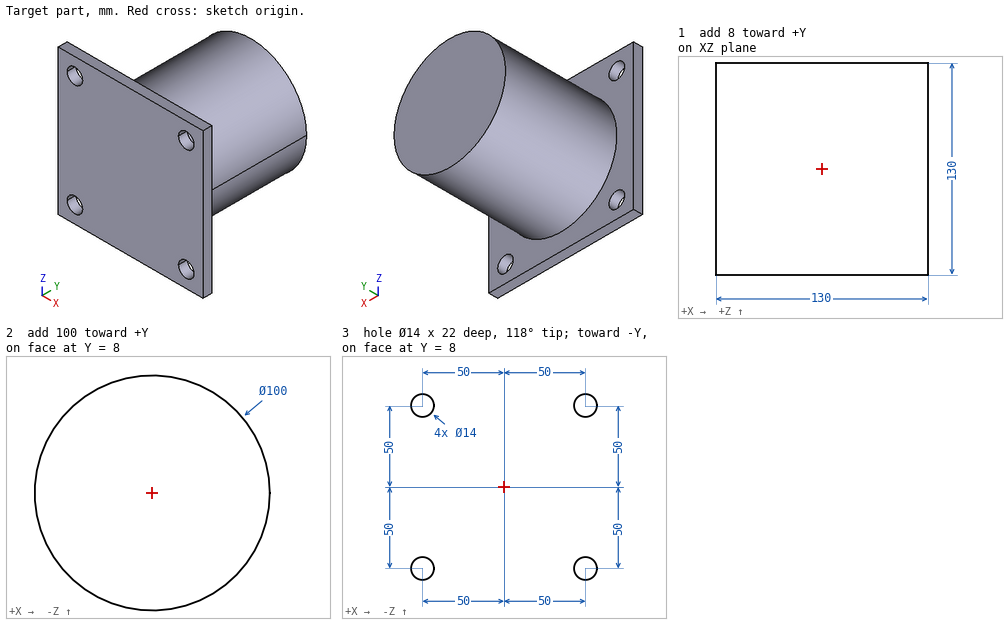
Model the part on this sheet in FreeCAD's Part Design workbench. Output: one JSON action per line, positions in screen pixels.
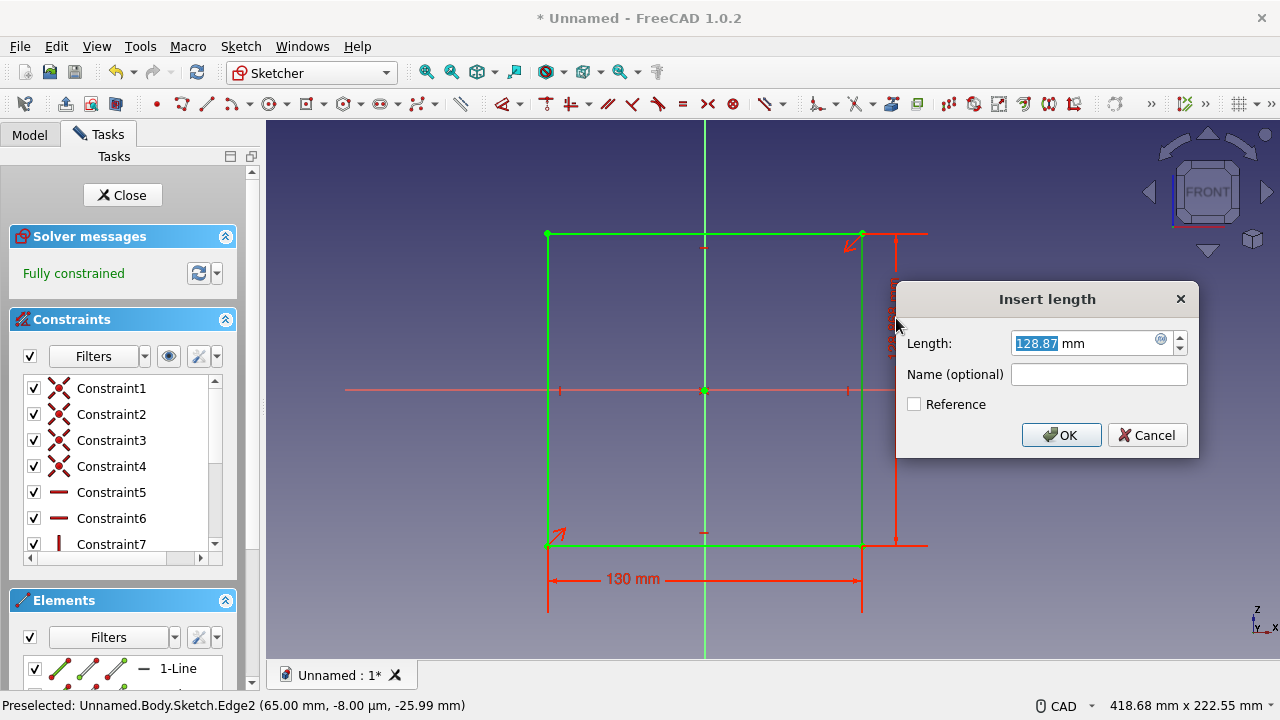
{"action": "type", "text": "130"}
{"action": "key", "text": "Return"}
{"action": "key", "text": "Escape"}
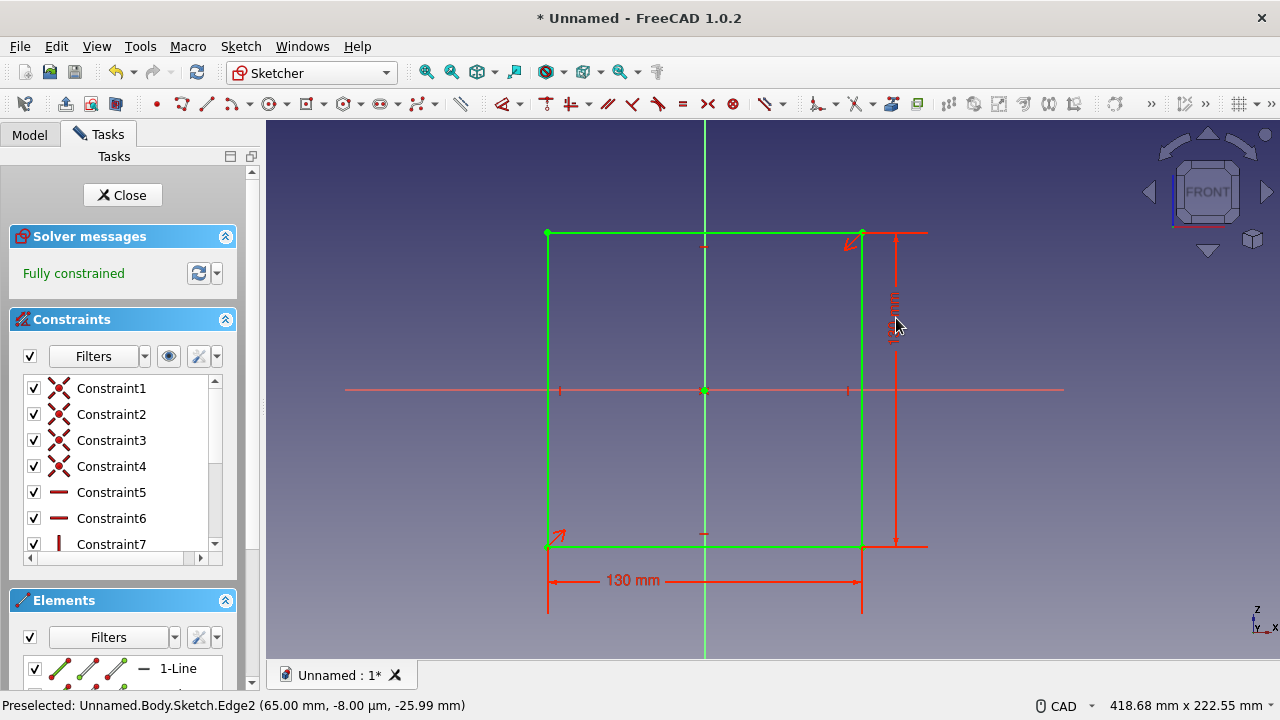
{"action": "left_click", "coordinate": [123, 195]}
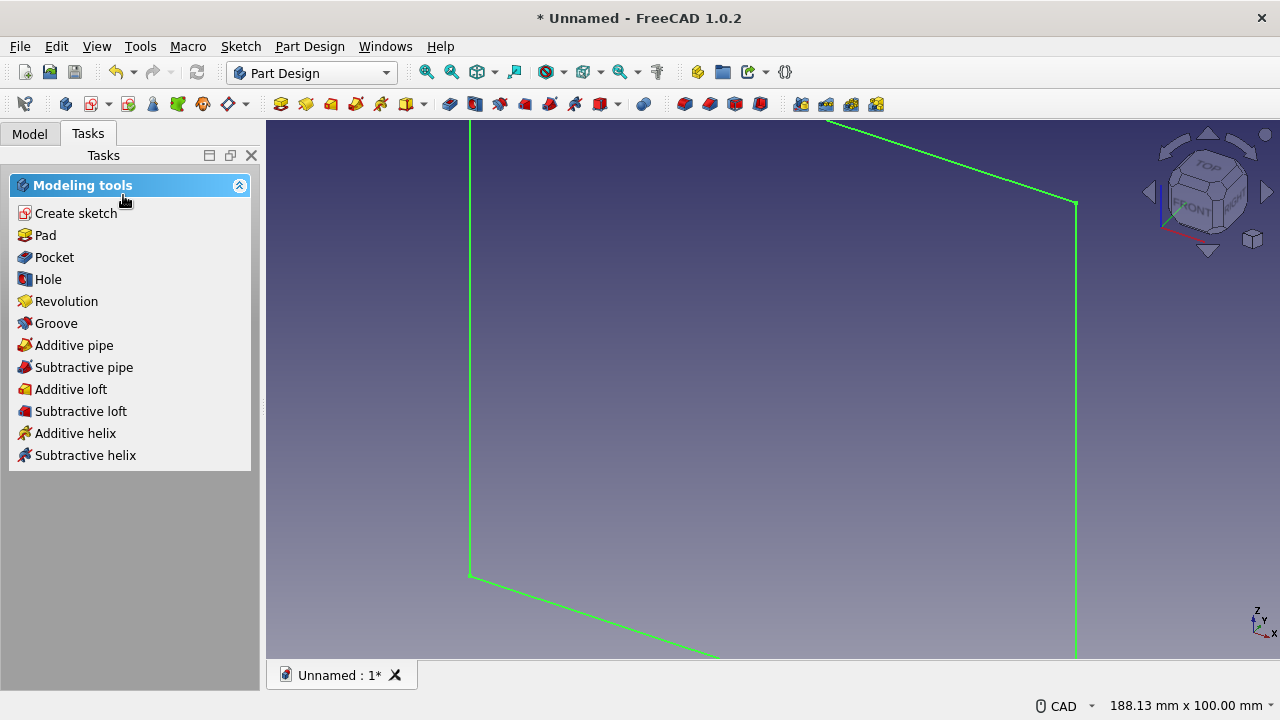
{"action": "left_click", "coordinate": [281, 104]}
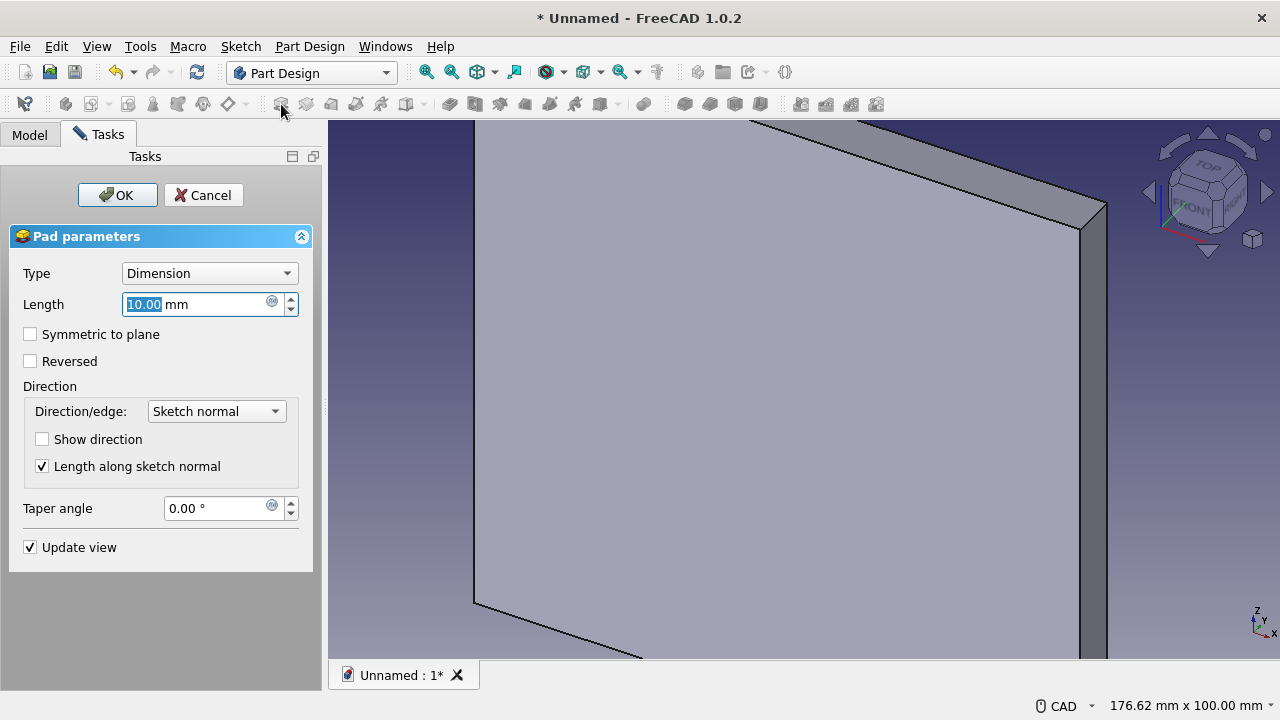
{"action": "type", "text": "8"}
{"action": "key", "text": "Tab"}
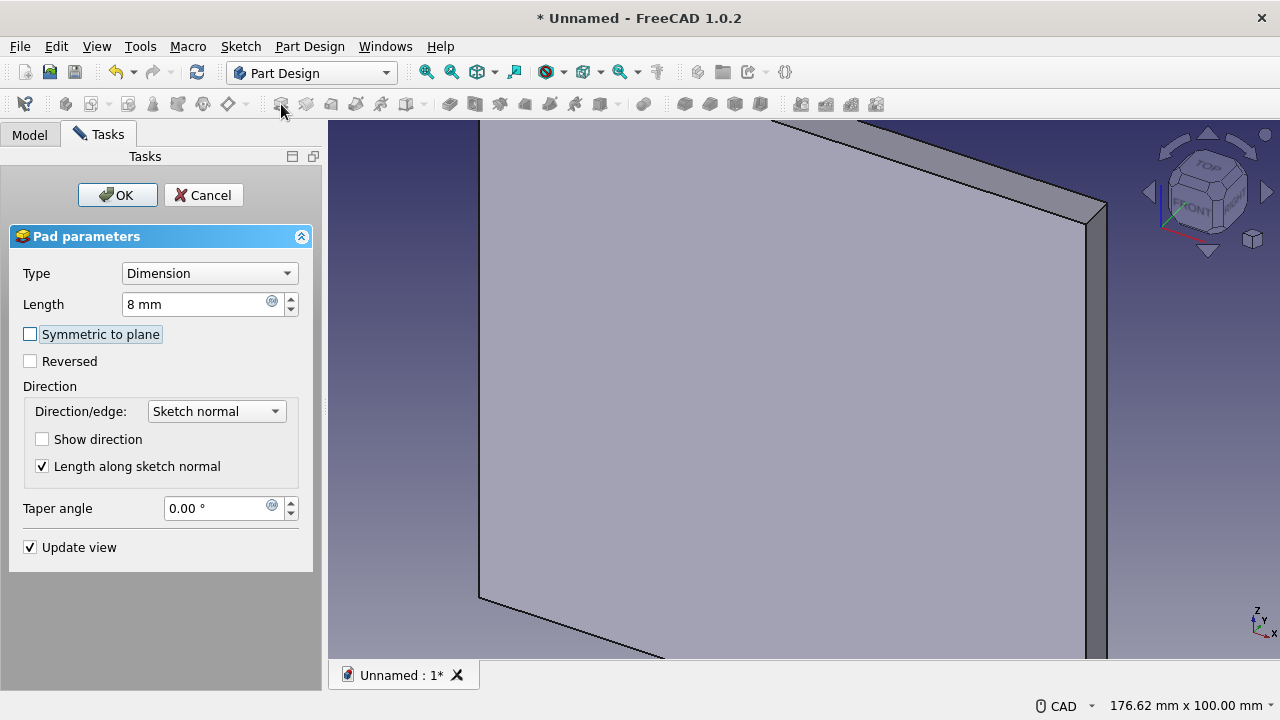
{"action": "left_click", "coordinate": [31, 361]}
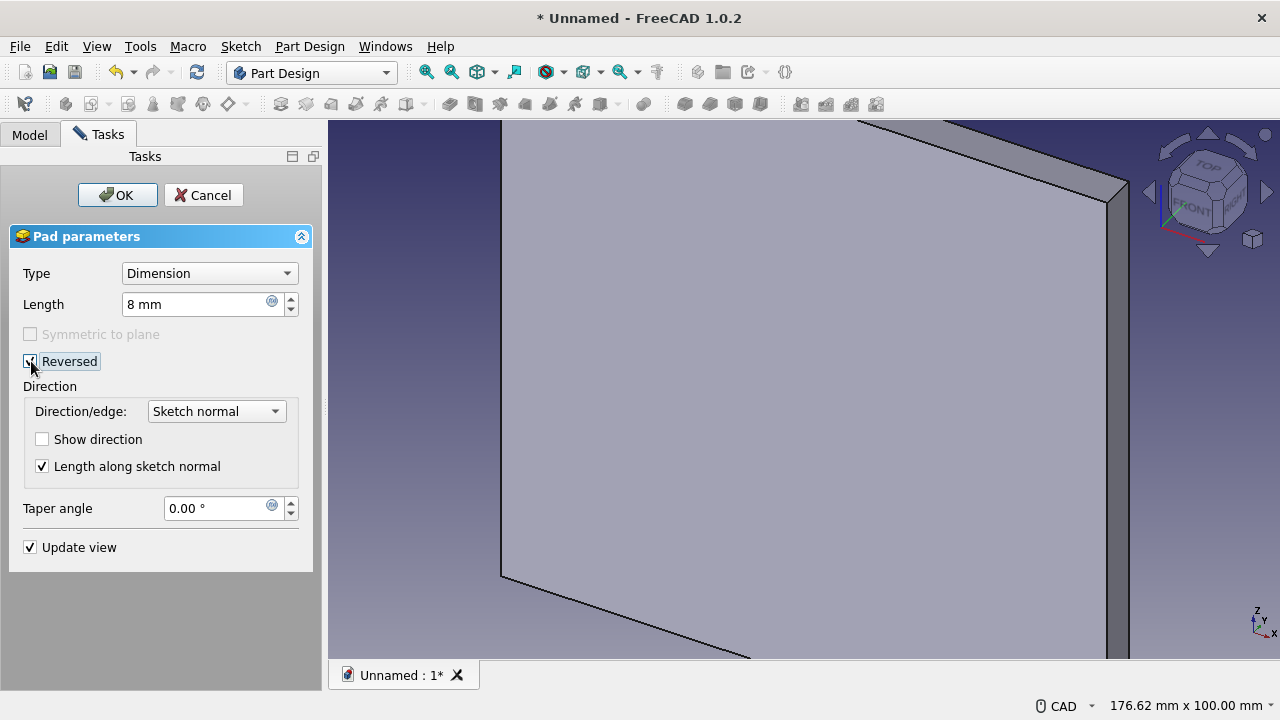
{"action": "left_click", "coordinate": [118, 195]}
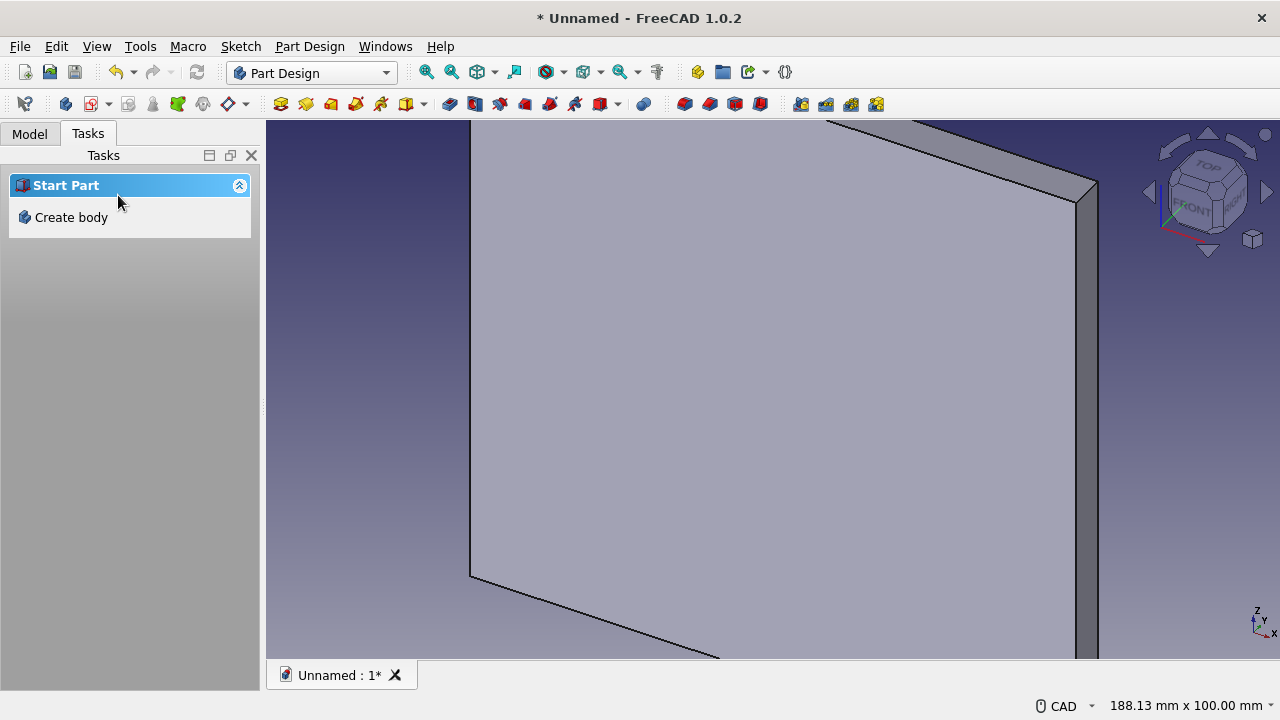
{"action": "key", "text": "v f"}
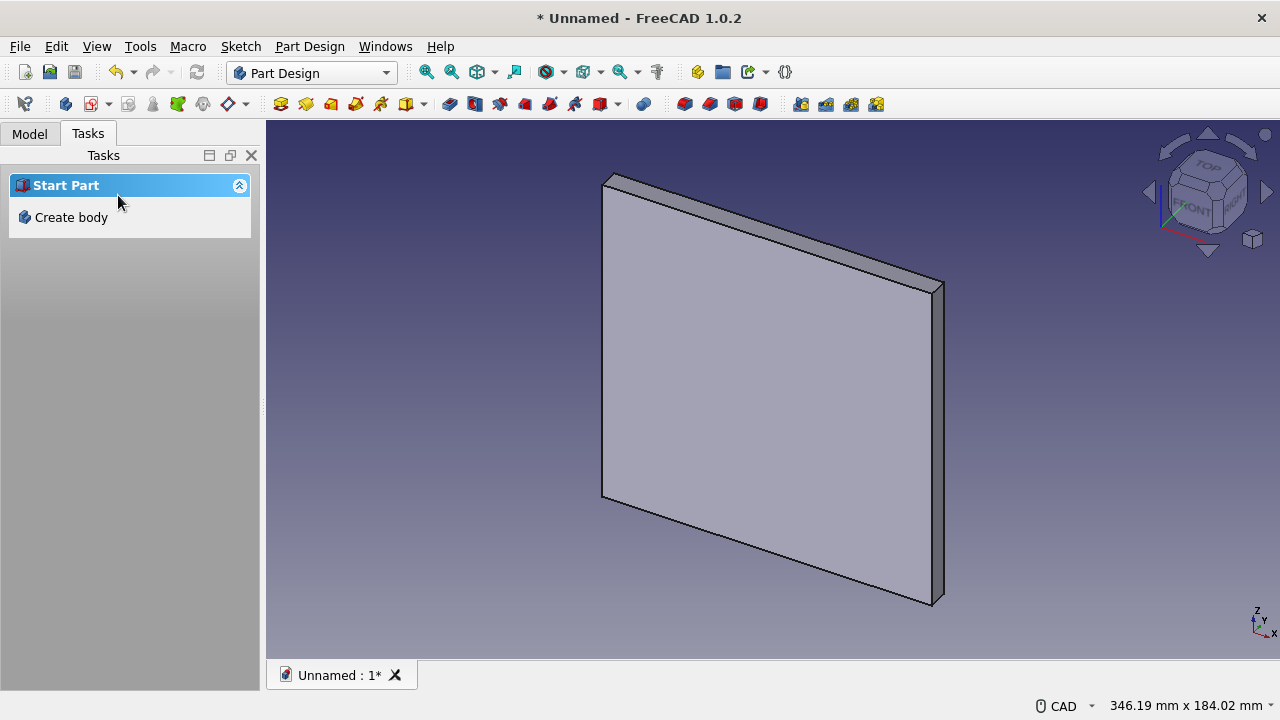
{"action": "key", "text": "4"}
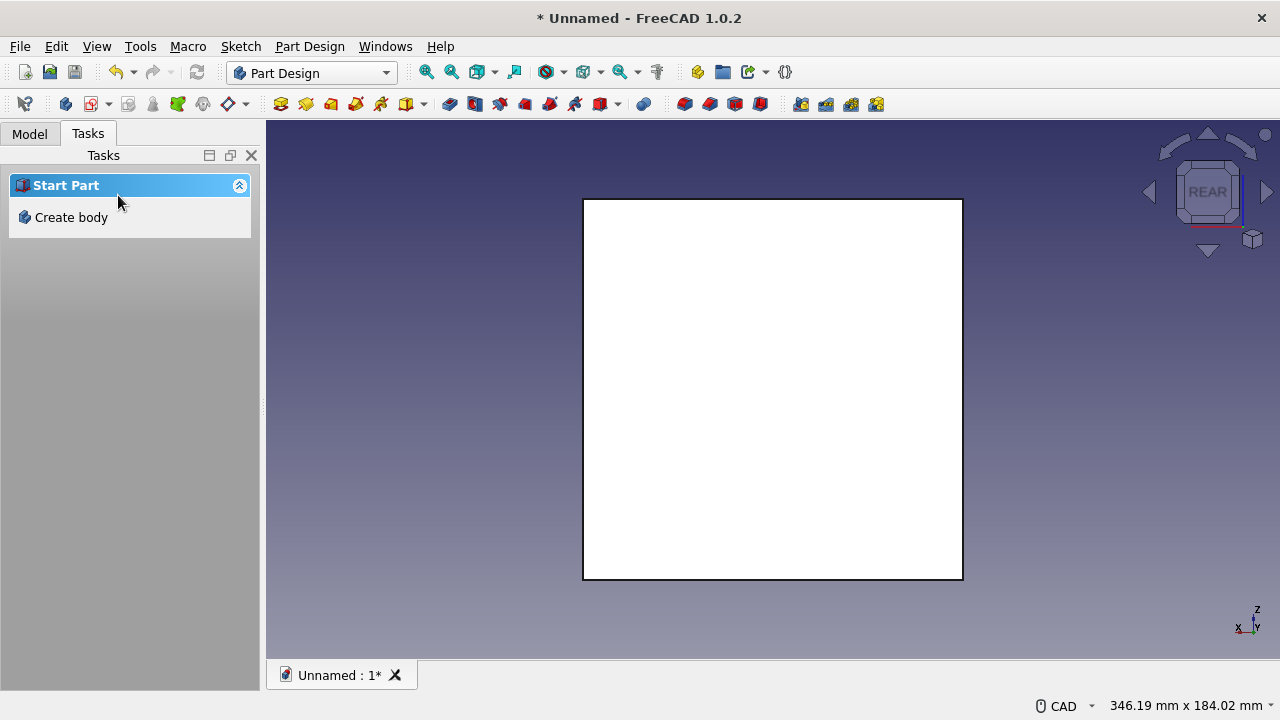
{"action": "left_click", "coordinate": [773, 389]}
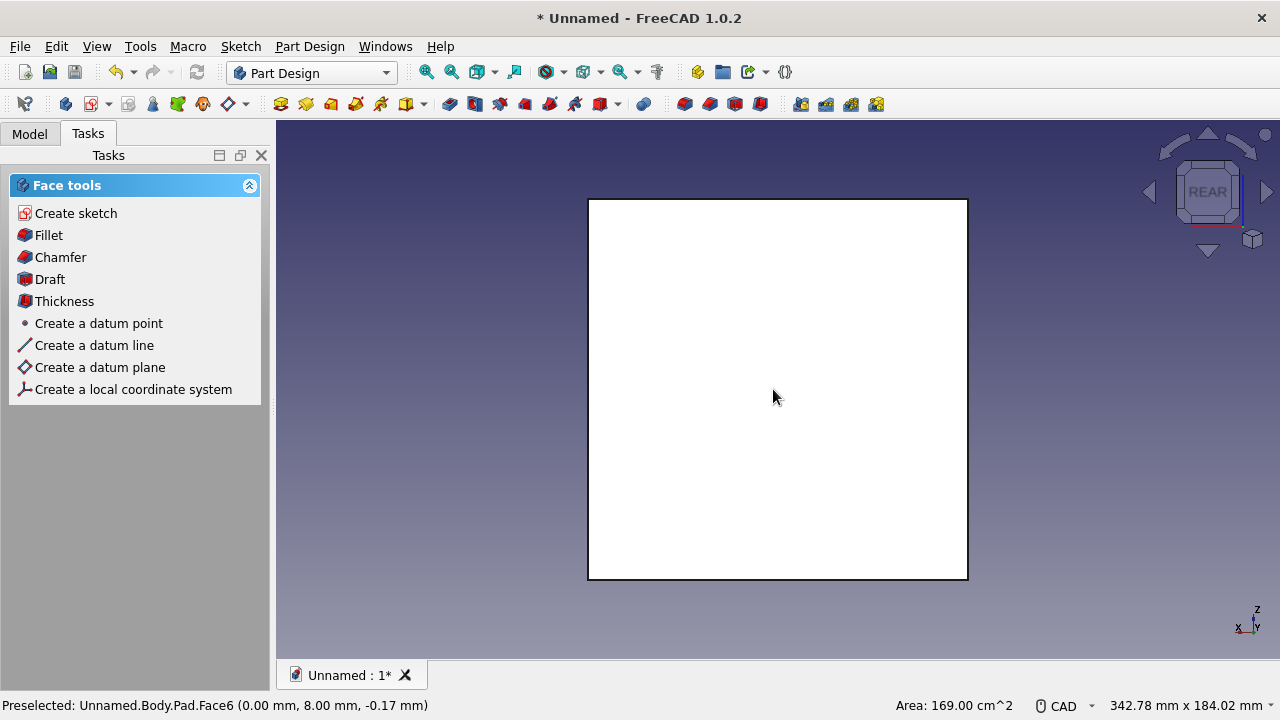
{"action": "left_click", "coordinate": [90, 104]}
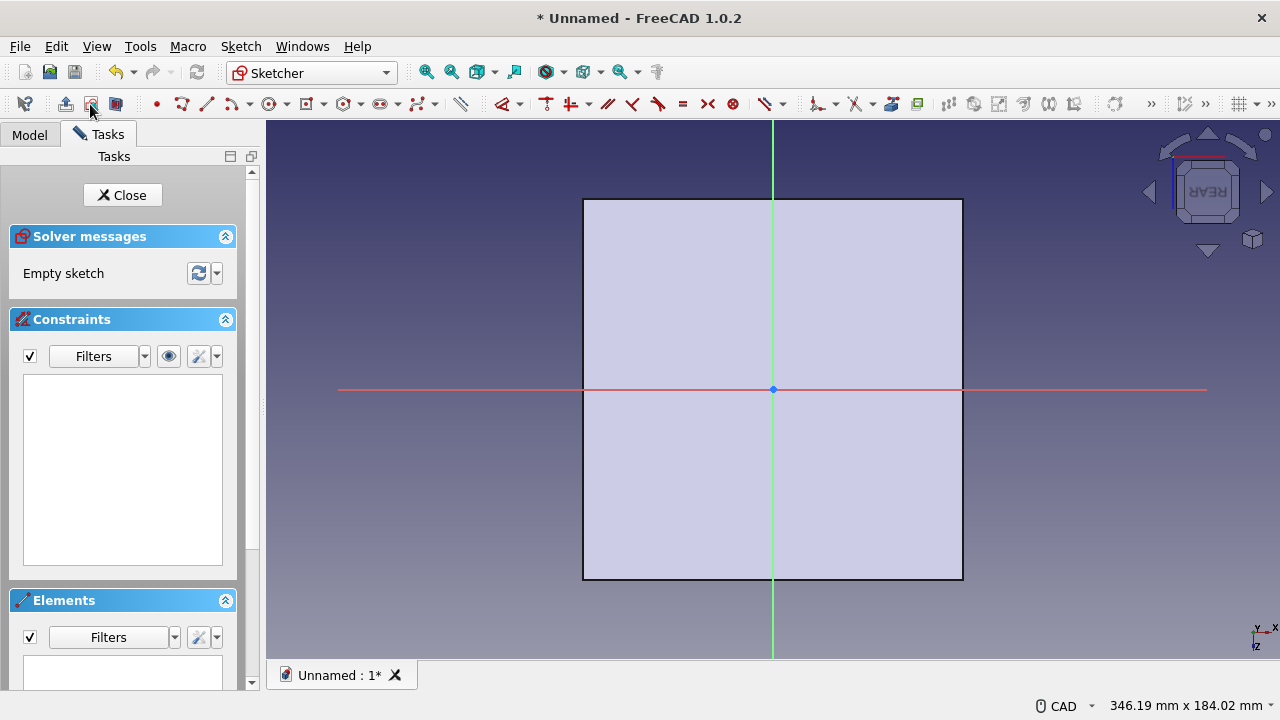
{"action": "left_click", "coordinate": [268, 104]}